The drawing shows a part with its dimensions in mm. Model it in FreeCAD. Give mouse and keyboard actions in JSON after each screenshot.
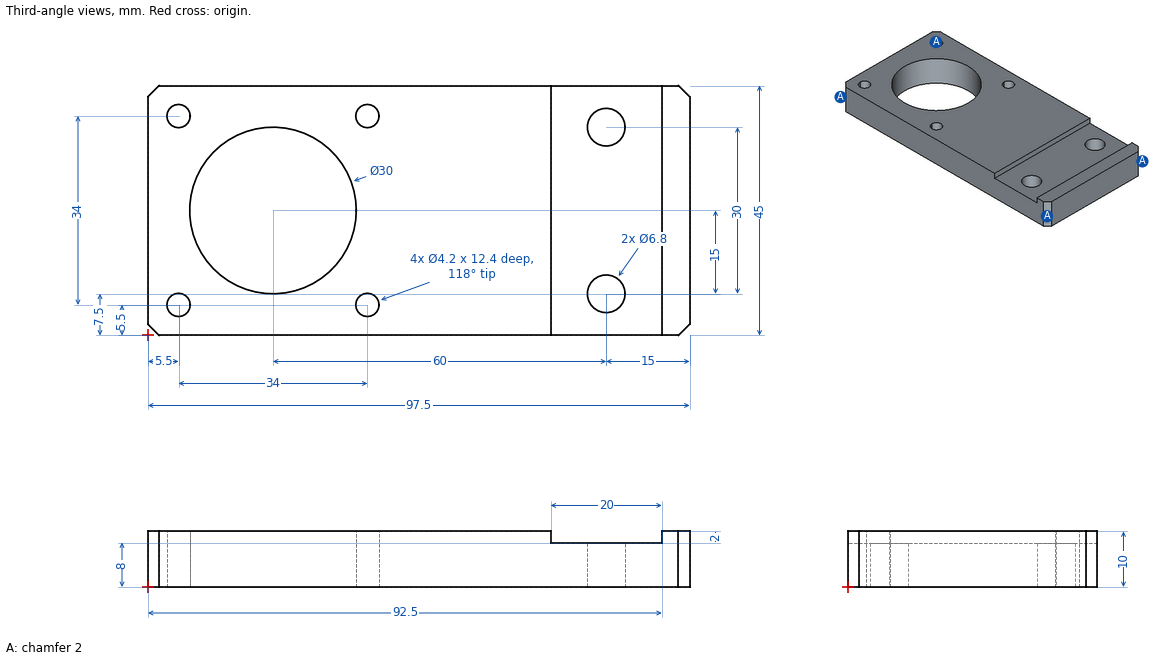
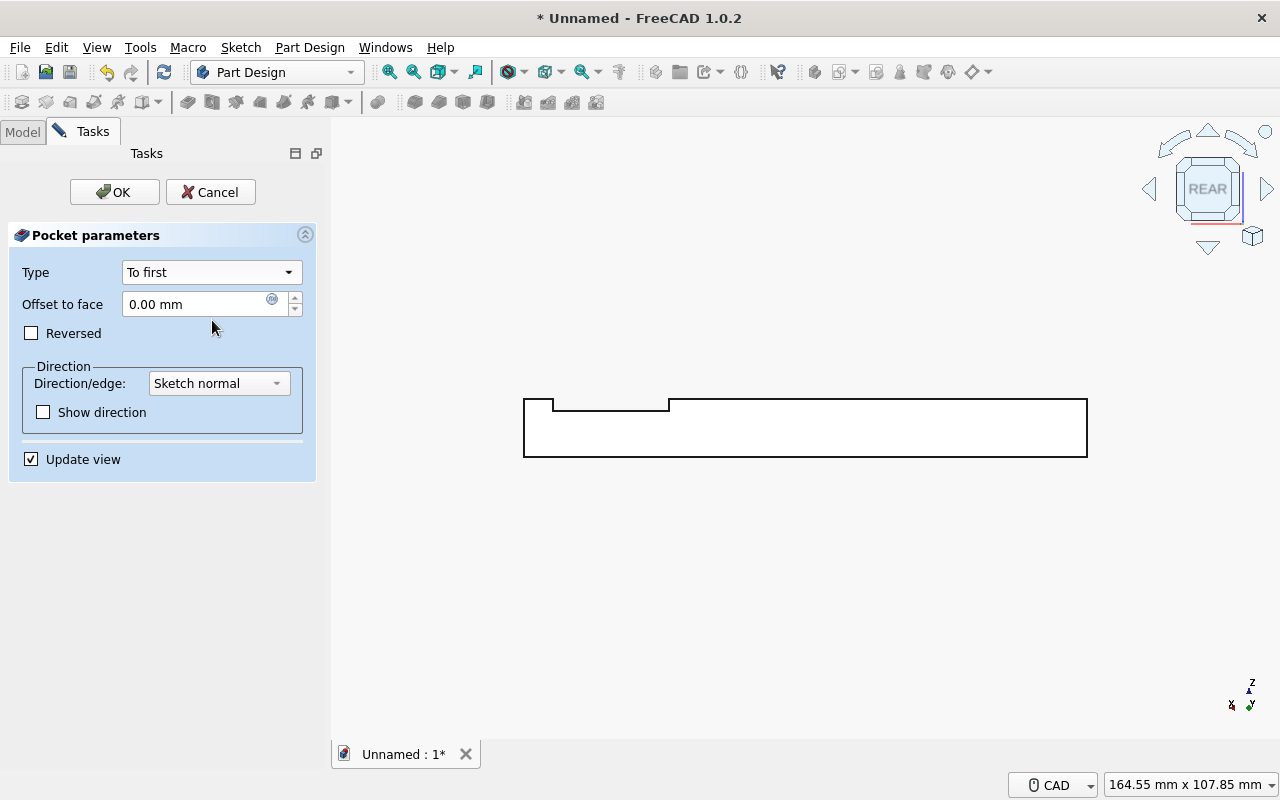
{"action": "left_click", "coordinate": [115, 192]}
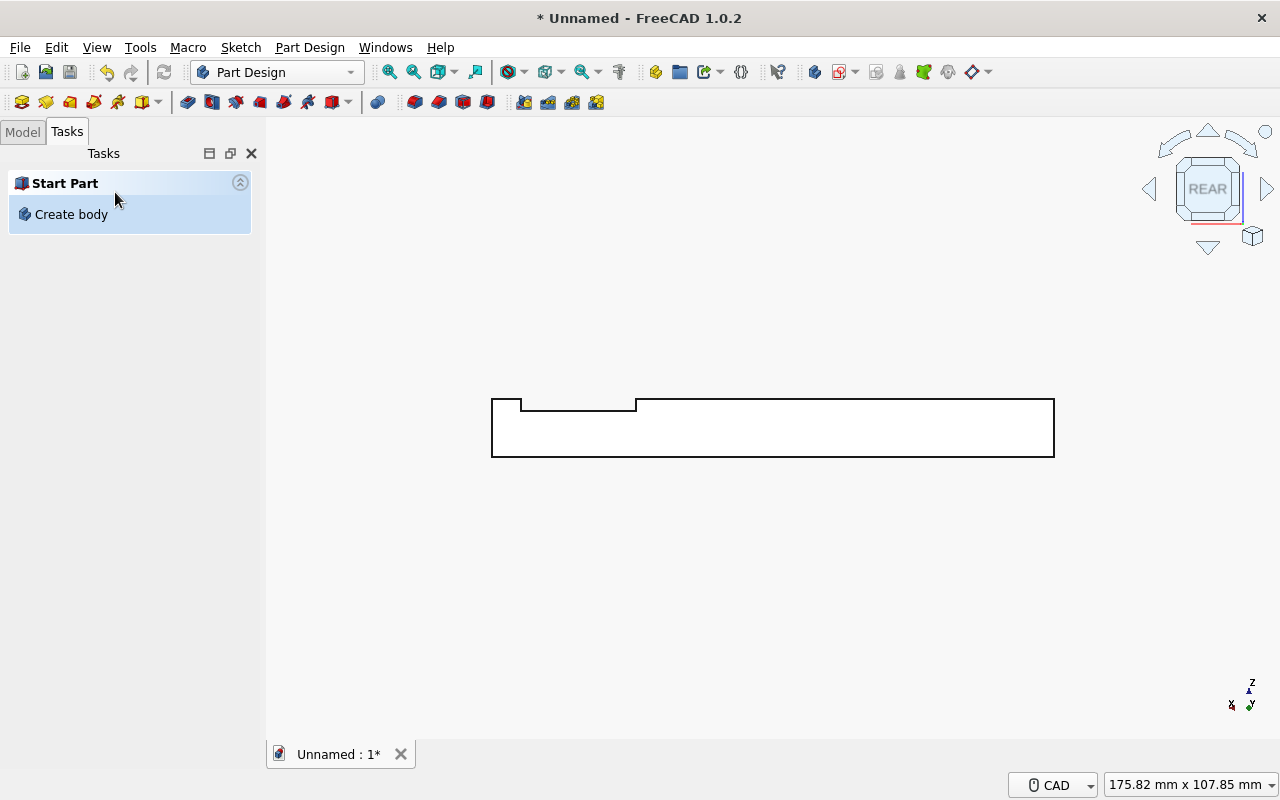
{"action": "key", "text": "5"}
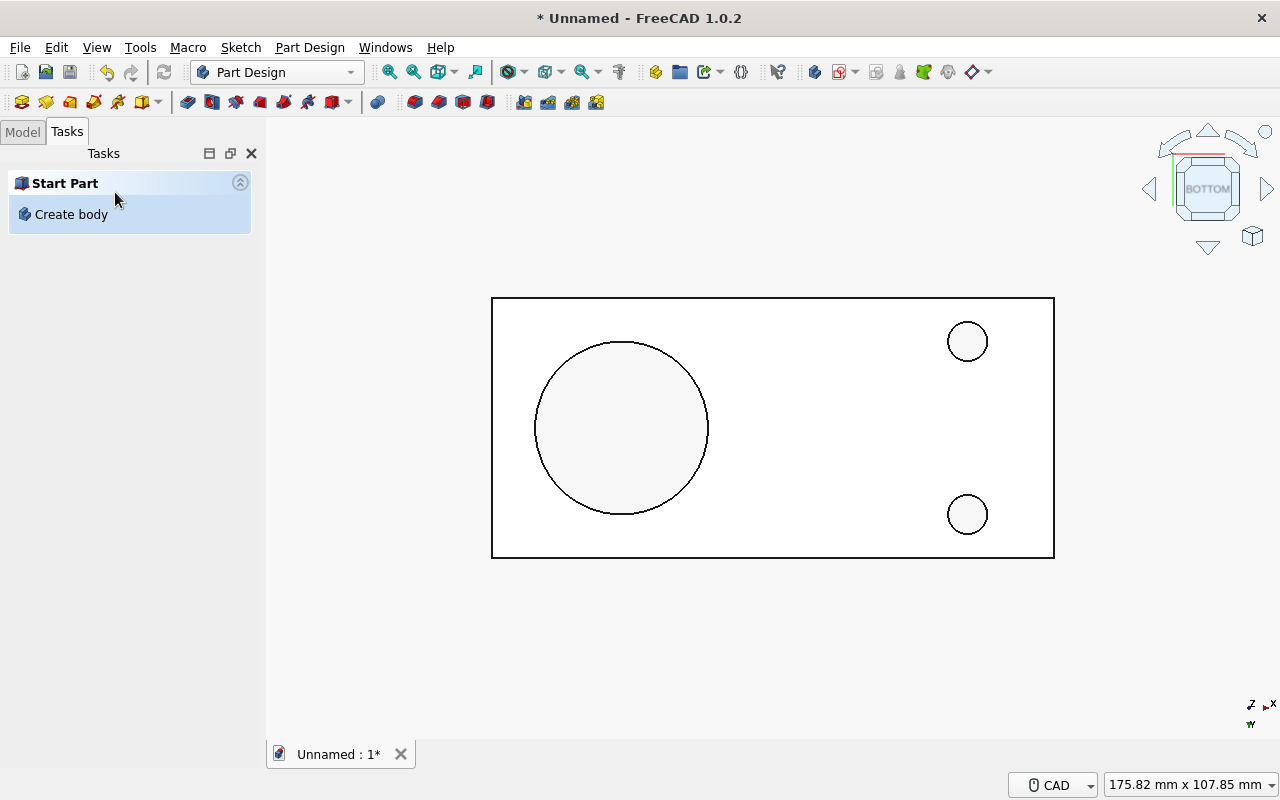
{"action": "left_click", "coordinate": [853, 427]}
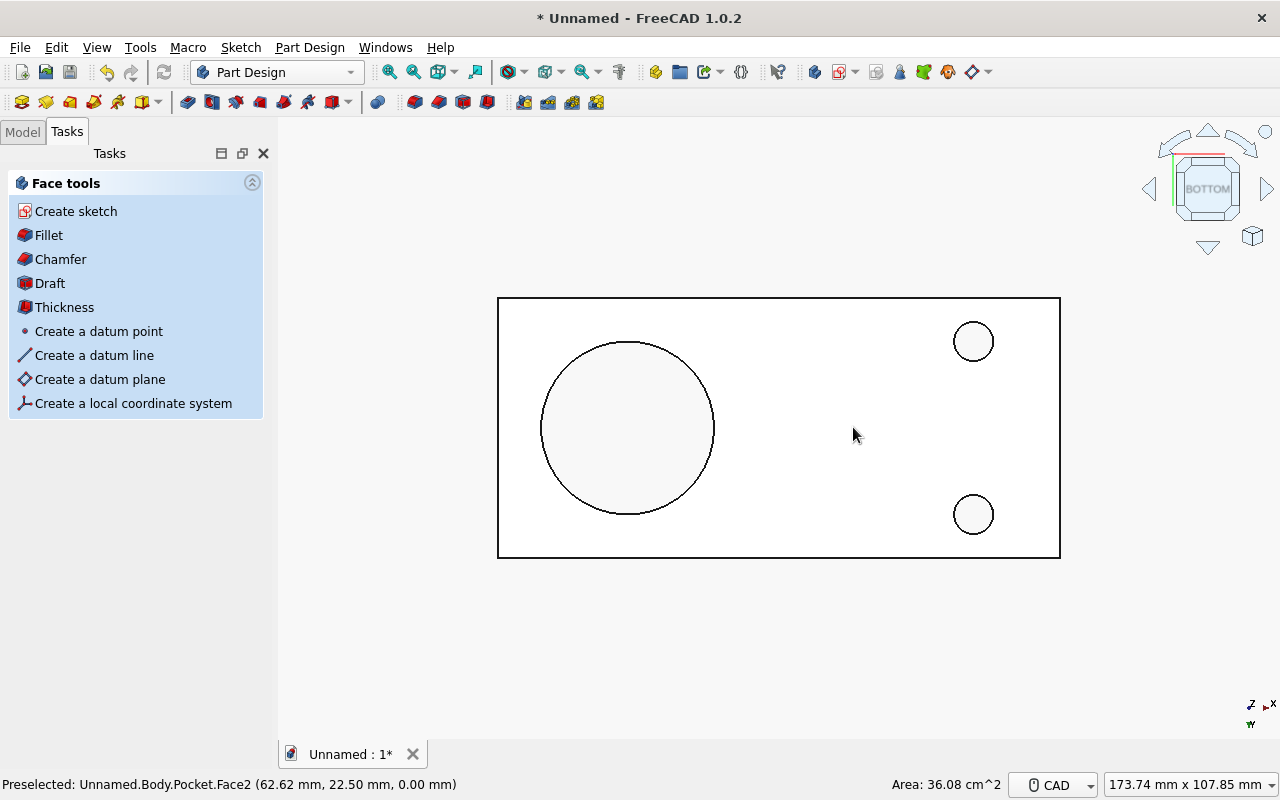
{"action": "left_click", "coordinate": [840, 72]}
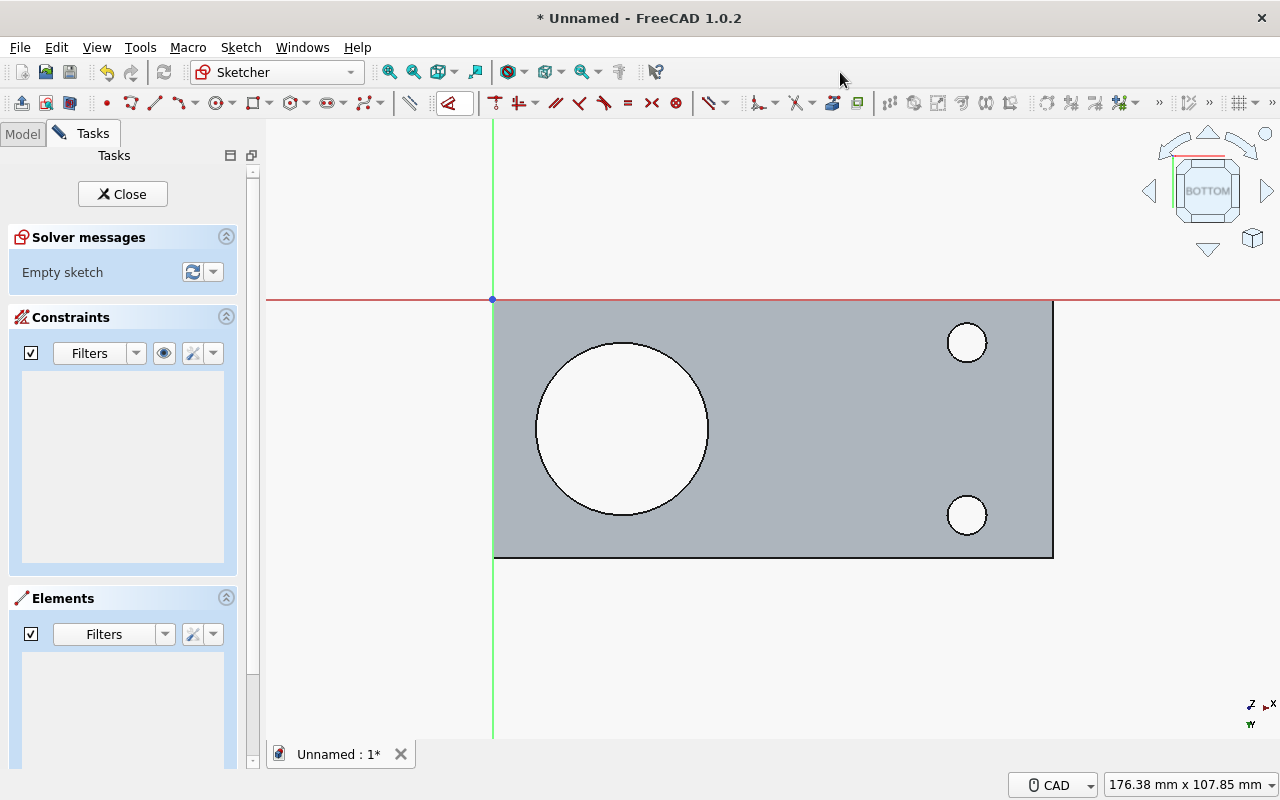
{"action": "scroll", "coordinate": [500, 407], "scroll_direction": "up", "scroll_amount": 3}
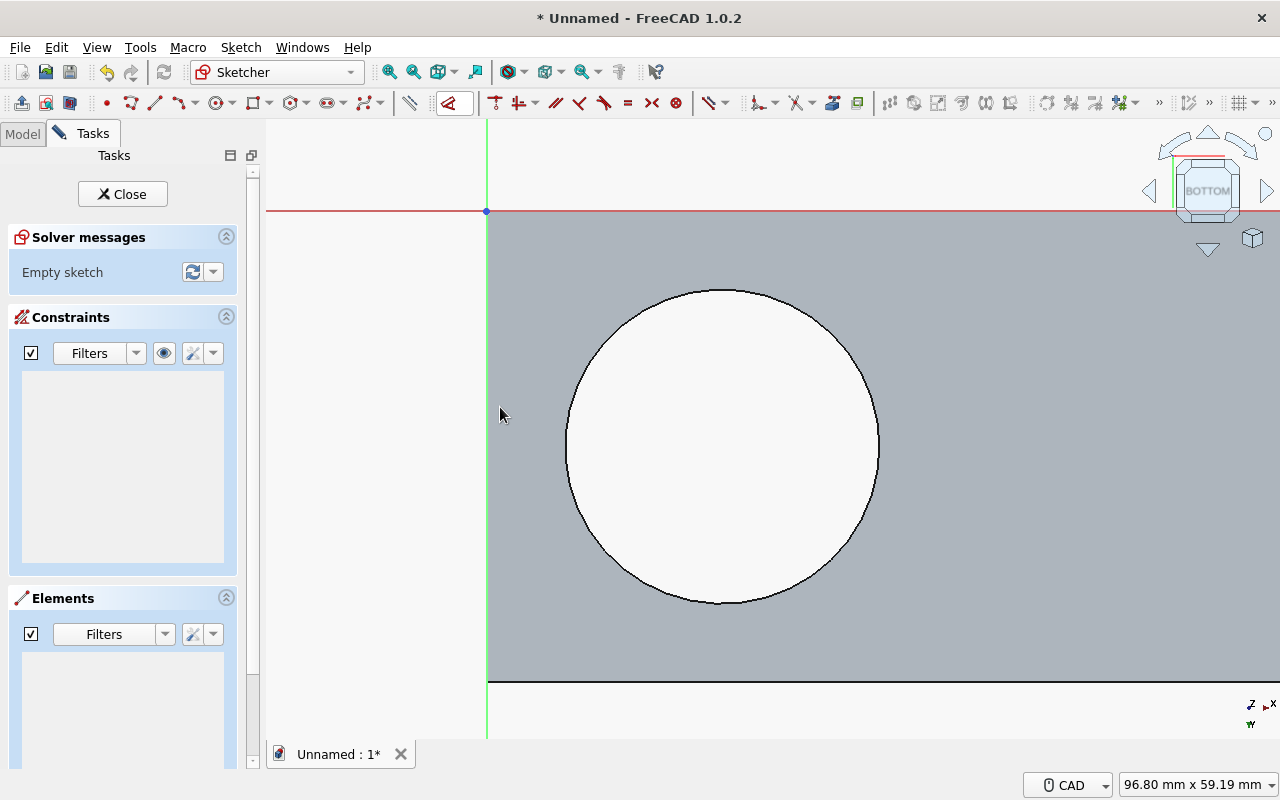
{"action": "key", "text": "g c"}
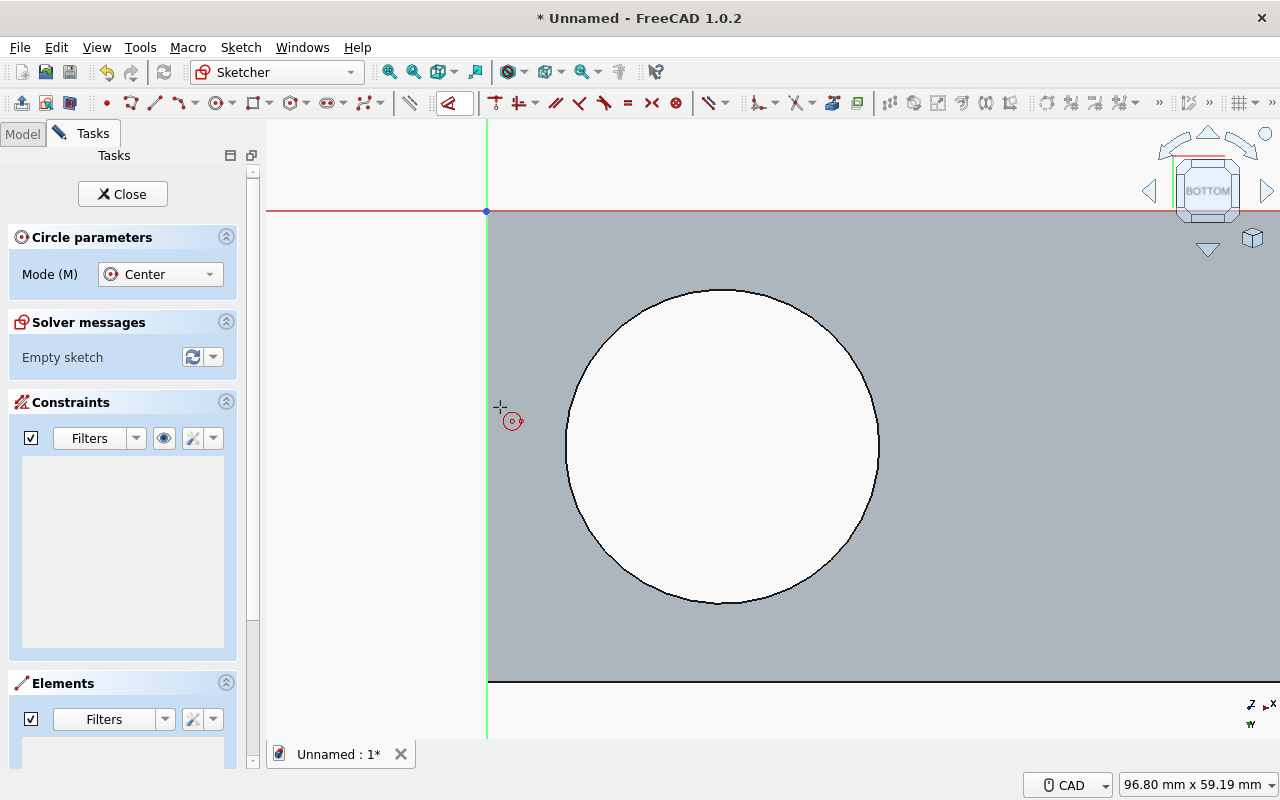
{"action": "left_click", "coordinate": [900, 269]}
{"action": "left_click", "coordinate": [916, 253]}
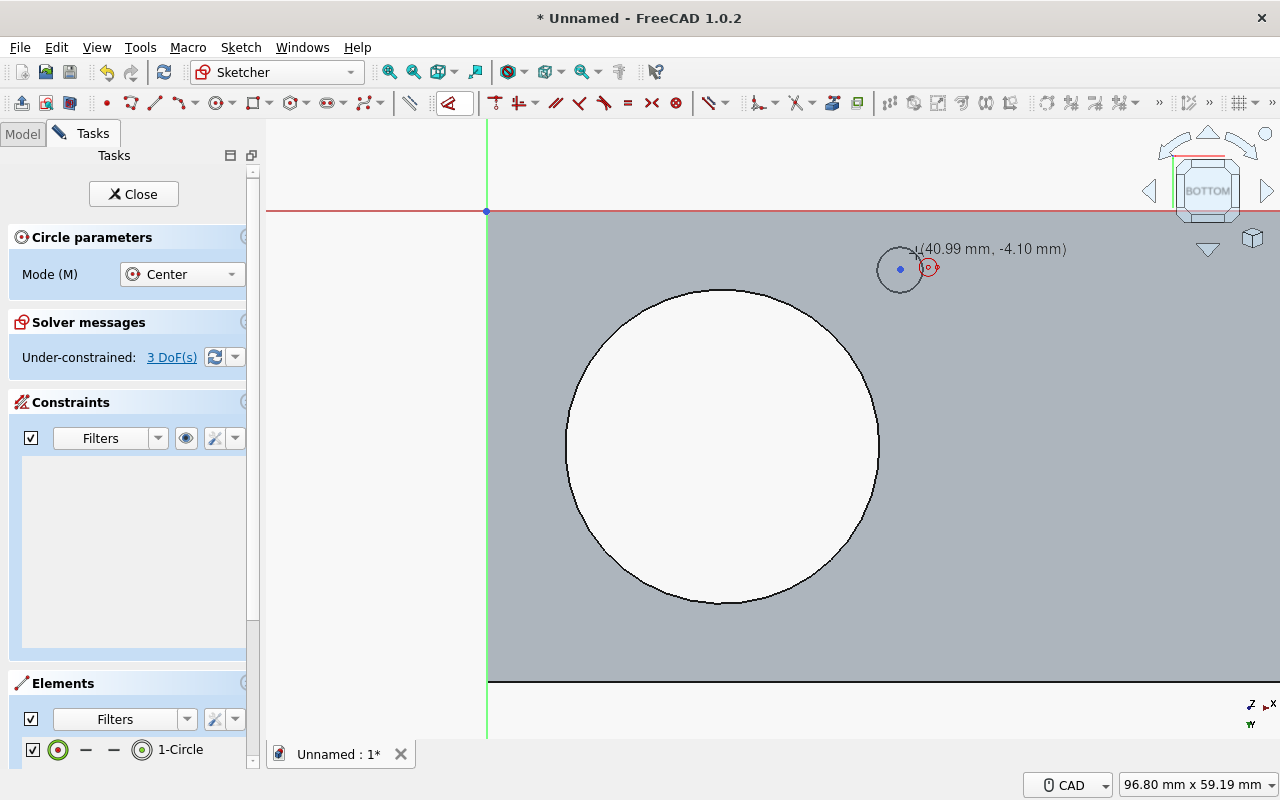
{"action": "left_click", "coordinate": [544, 269]}
{"action": "left_click", "coordinate": [560, 253]}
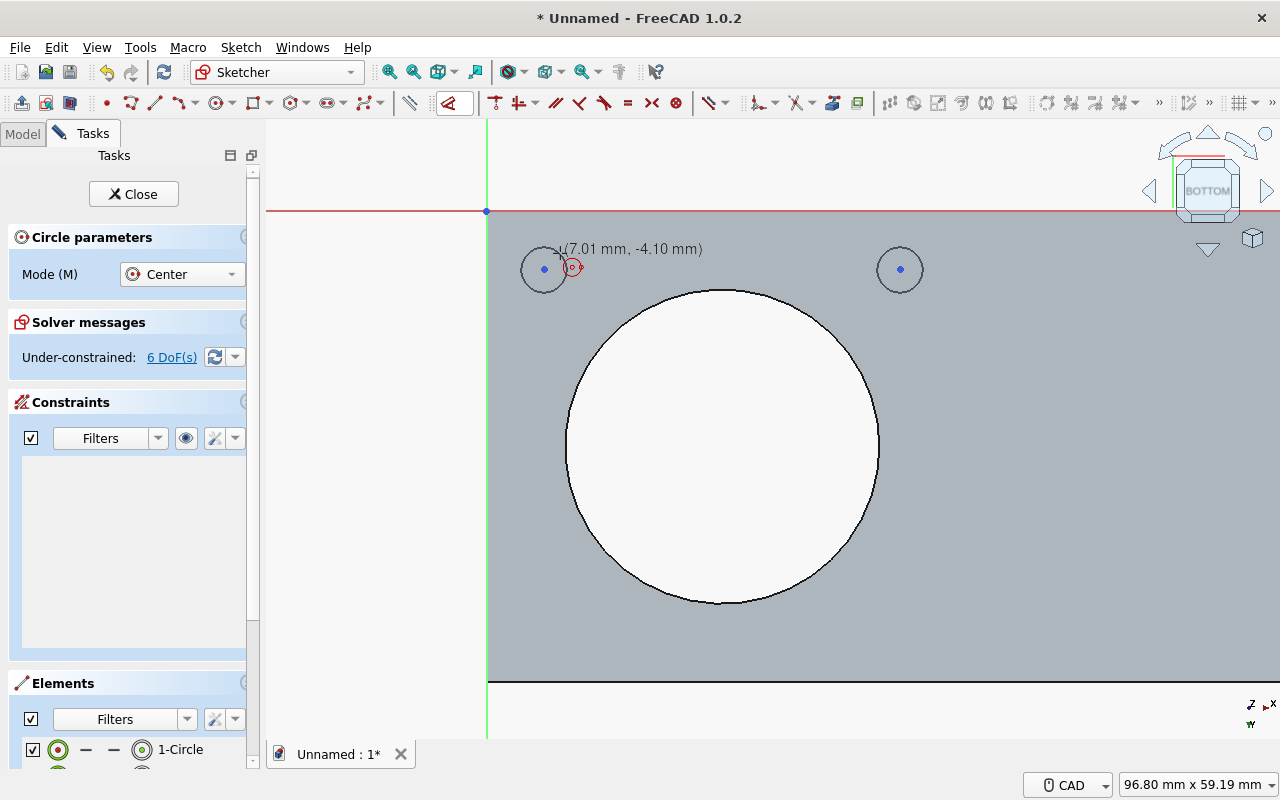
{"action": "left_click", "coordinate": [544, 625]}
{"action": "left_click", "coordinate": [560, 609]}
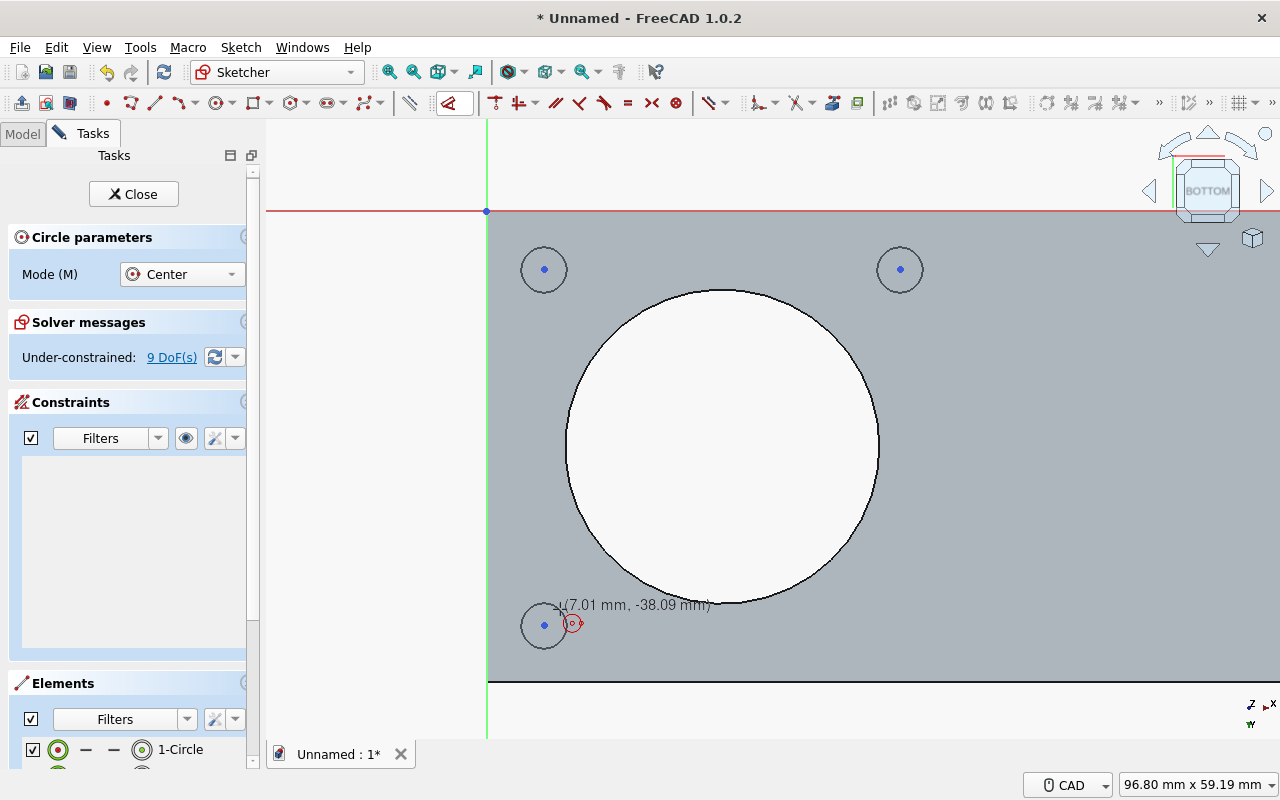
{"action": "left_click", "coordinate": [900, 625]}
{"action": "left_click", "coordinate": [916, 609]}
{"action": "key", "text": "Escape"}